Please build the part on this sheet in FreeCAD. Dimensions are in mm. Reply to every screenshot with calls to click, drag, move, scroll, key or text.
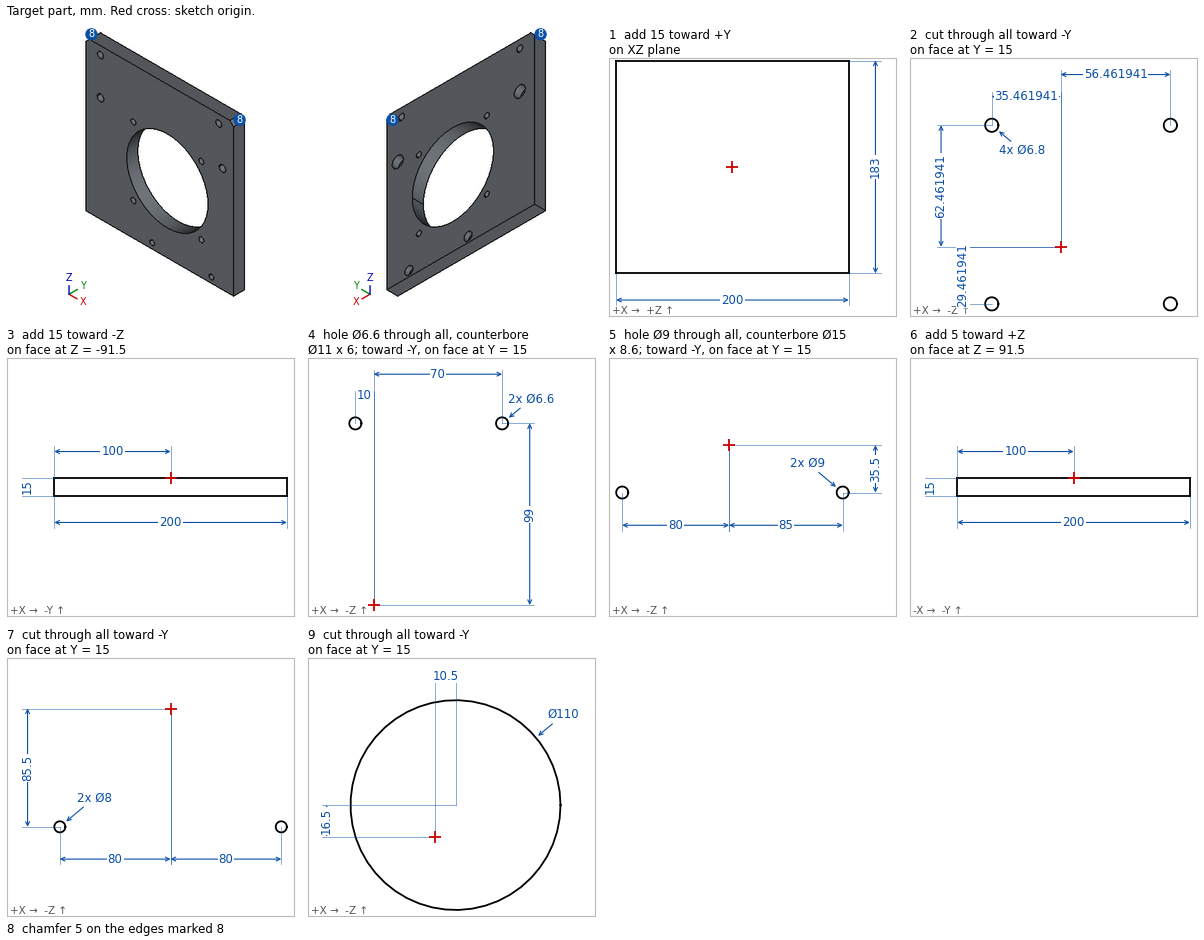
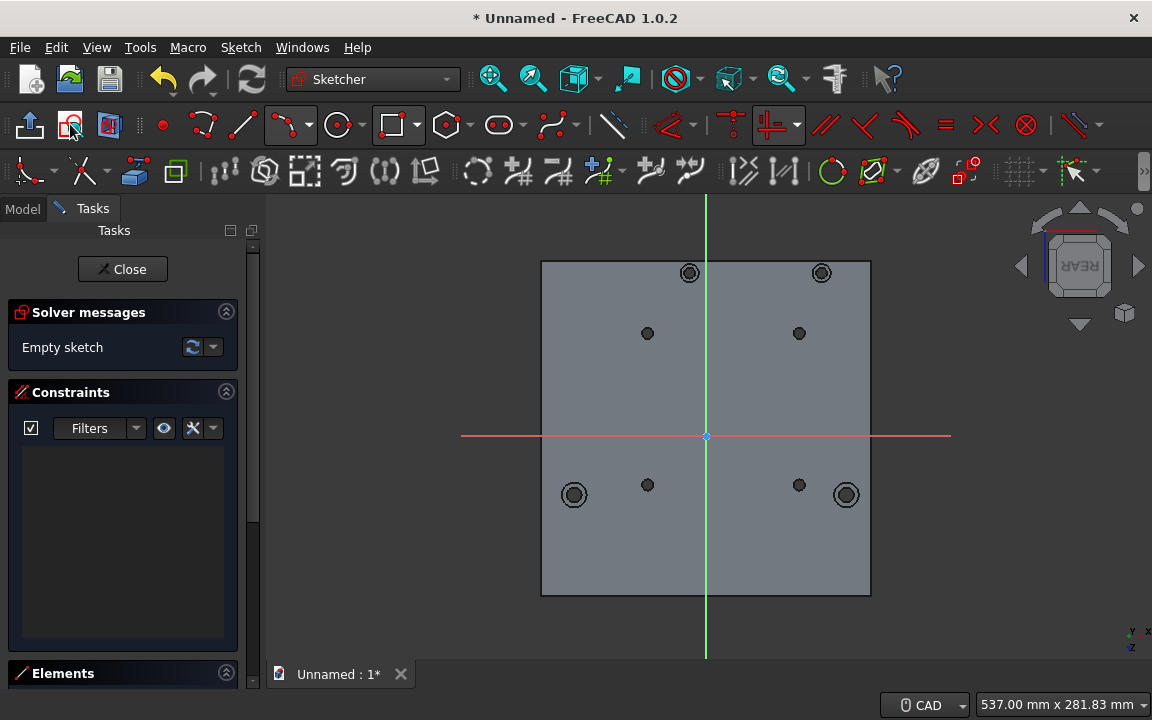
scroll(786, 612, up, 3)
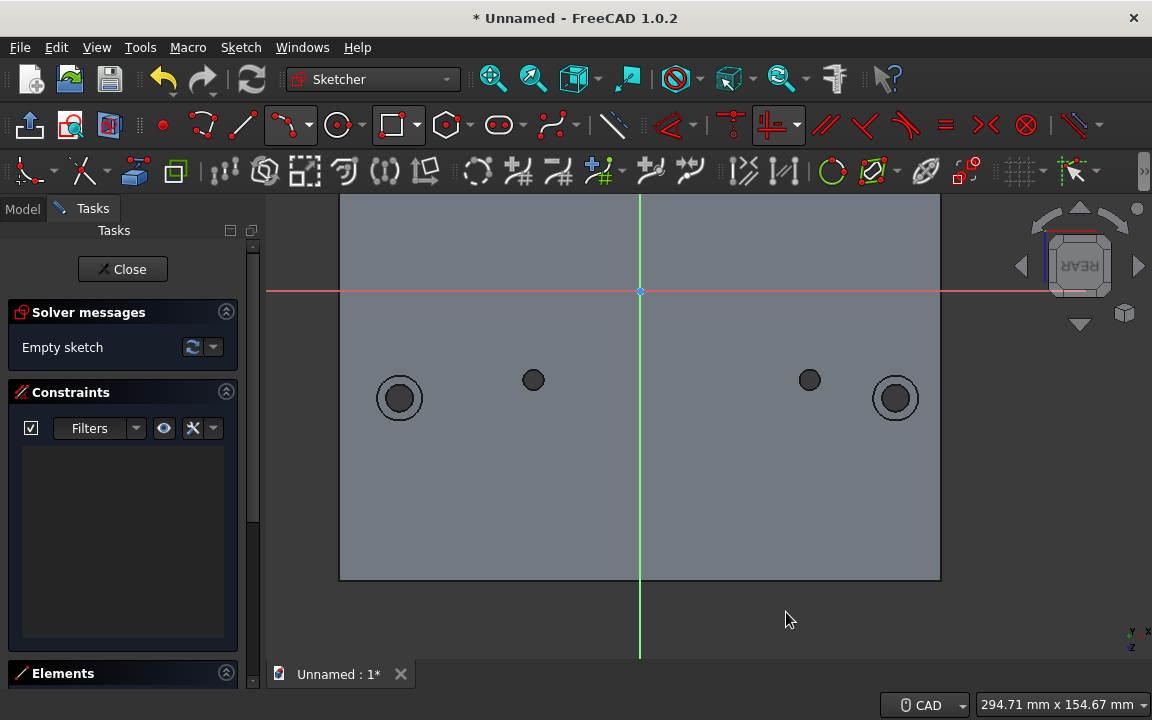
click(338, 126)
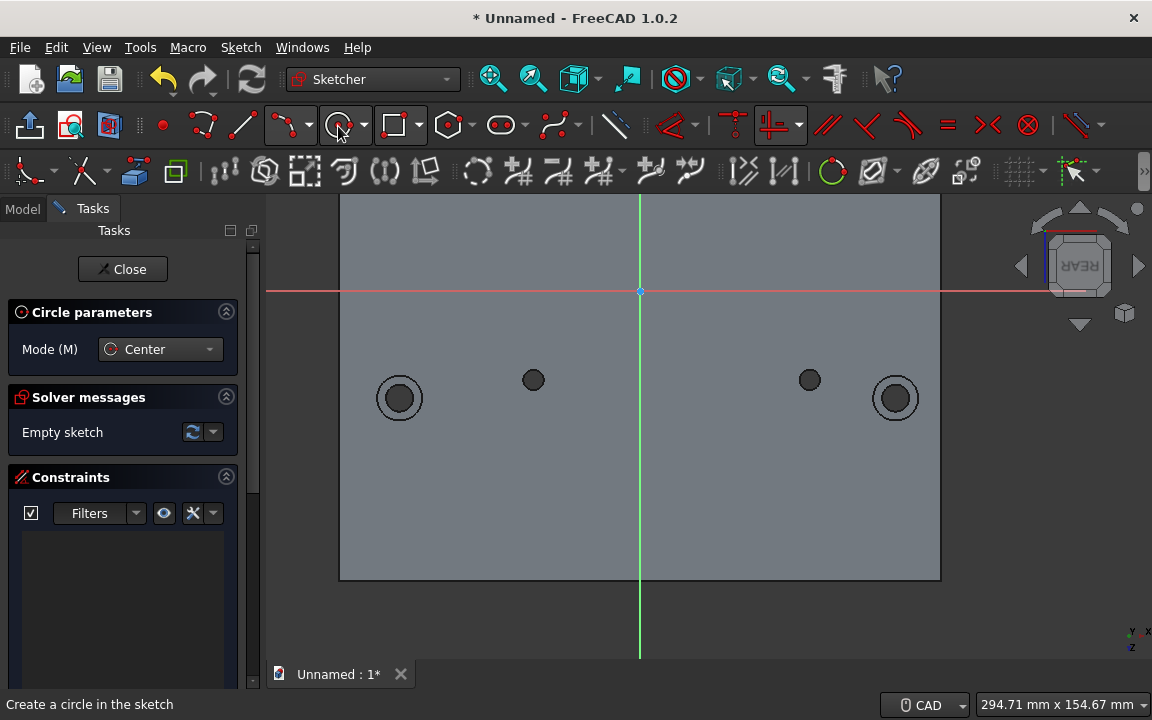
scroll(400, 548, up, 4)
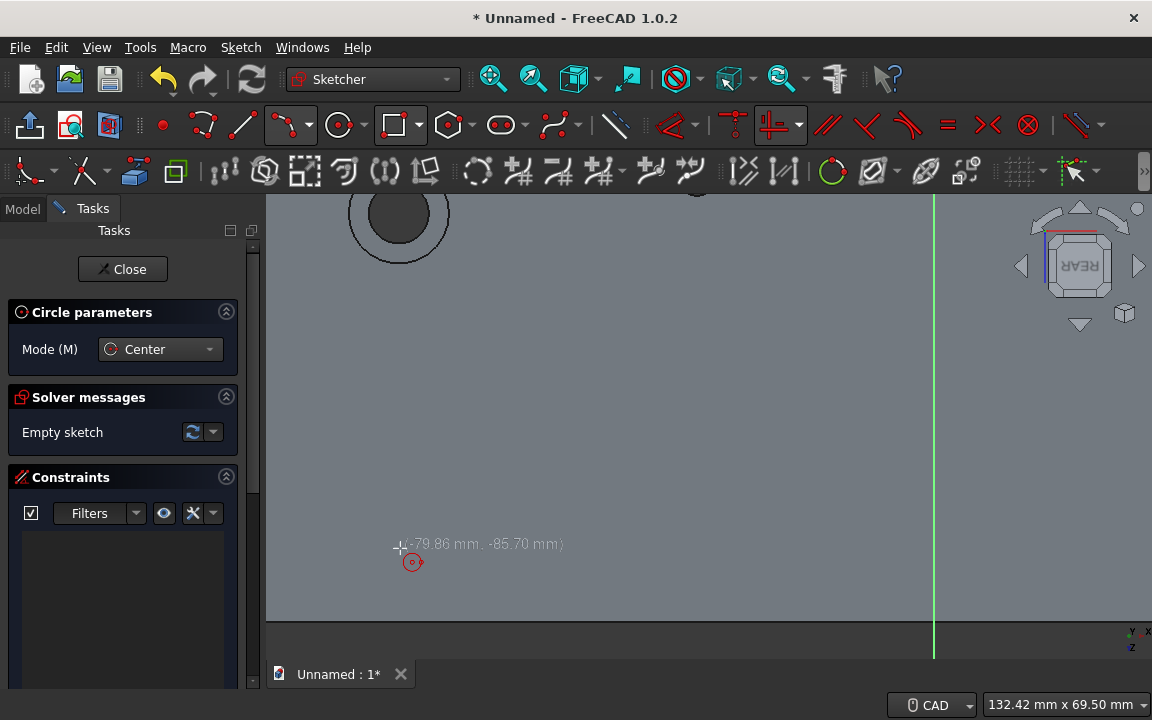
click(399, 548)
click(418, 529)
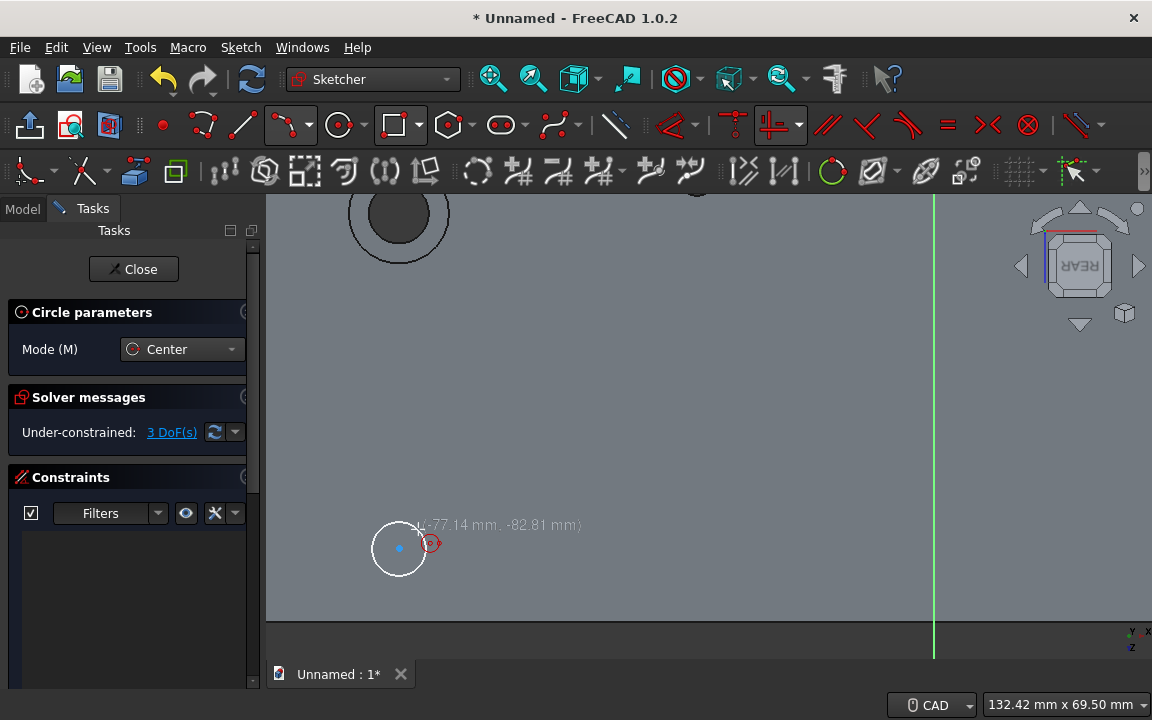
scroll(401, 550, down, 4)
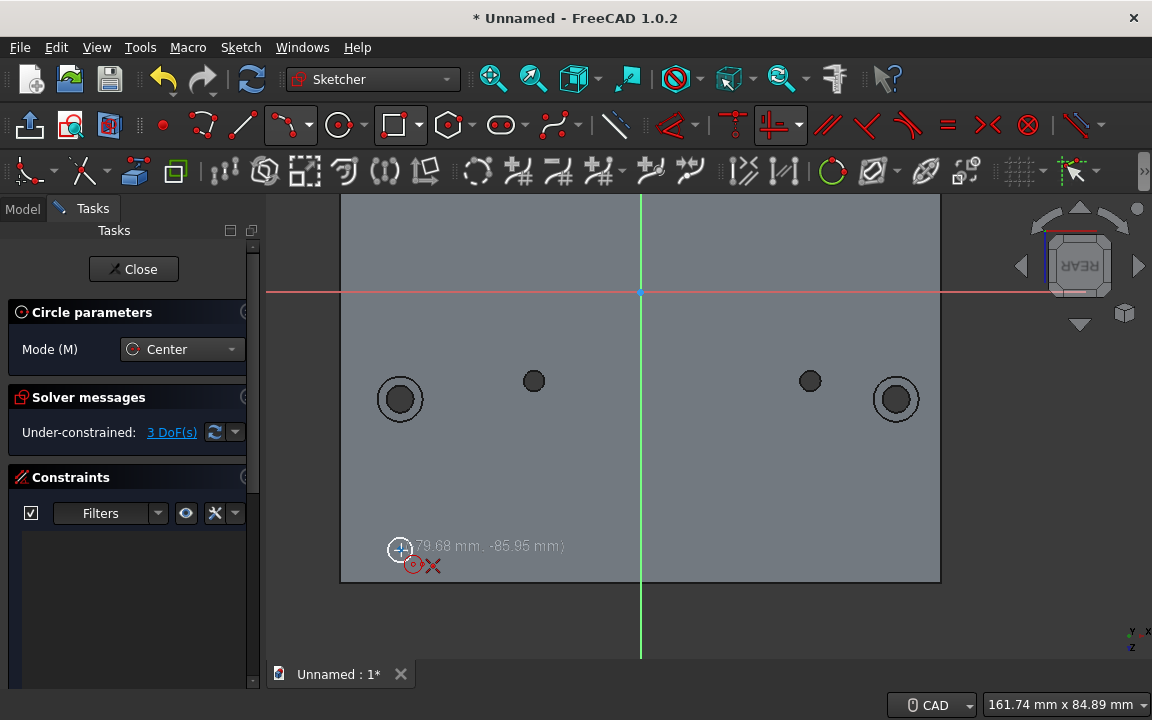
scroll(881, 550, up, 4)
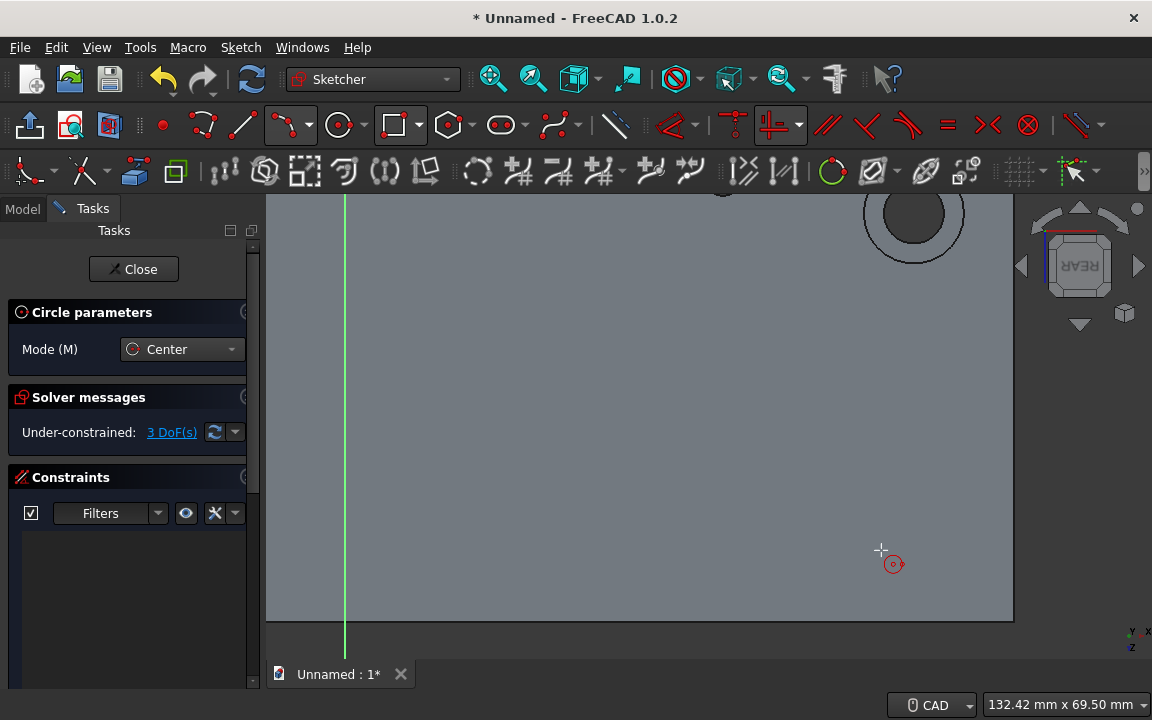
click(880, 548)
click(899, 529)
key(Escape)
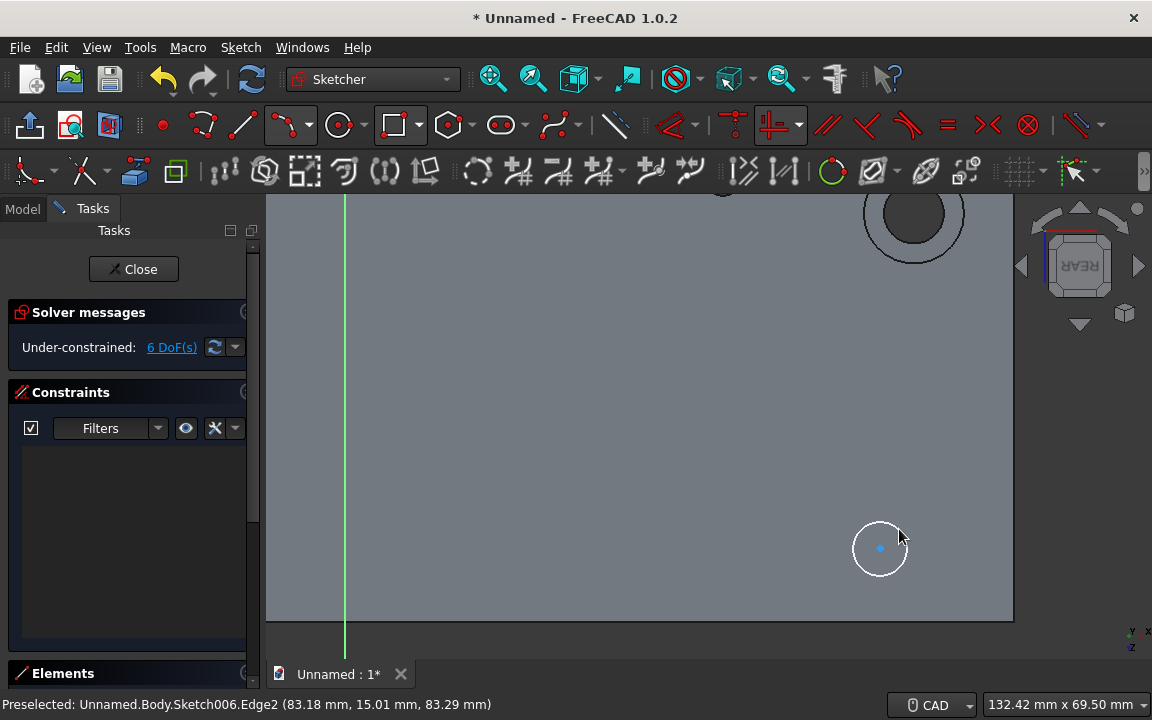
scroll(881, 550, down, 4)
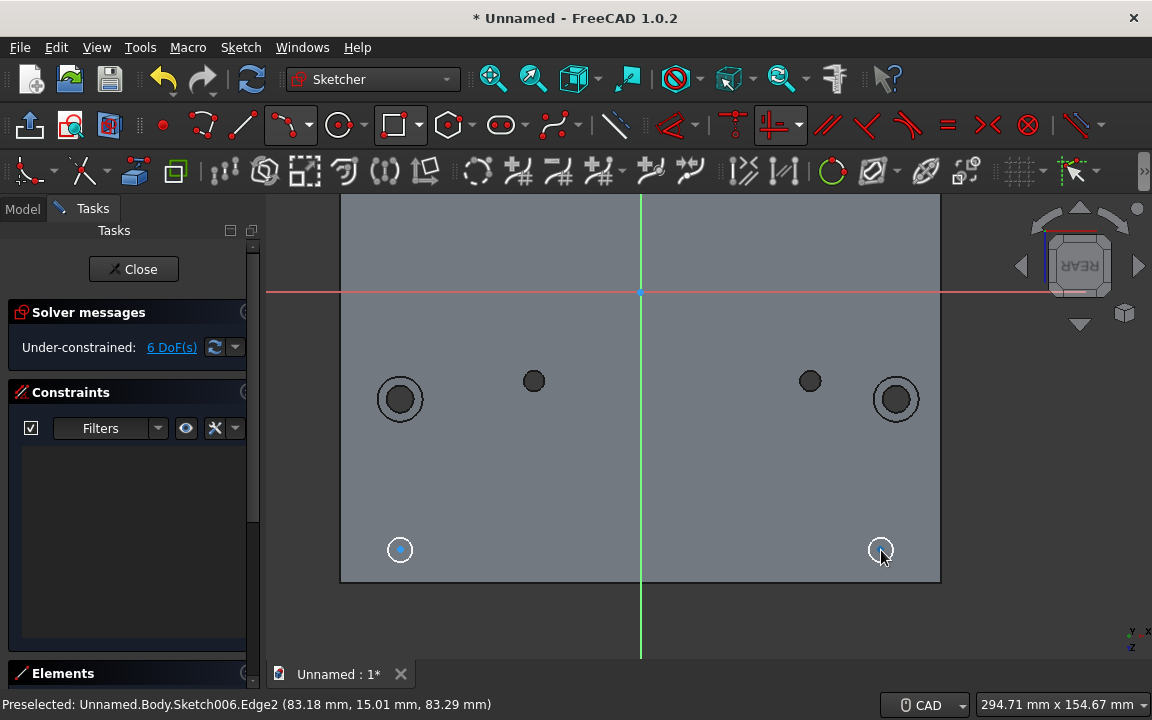
click(409, 541)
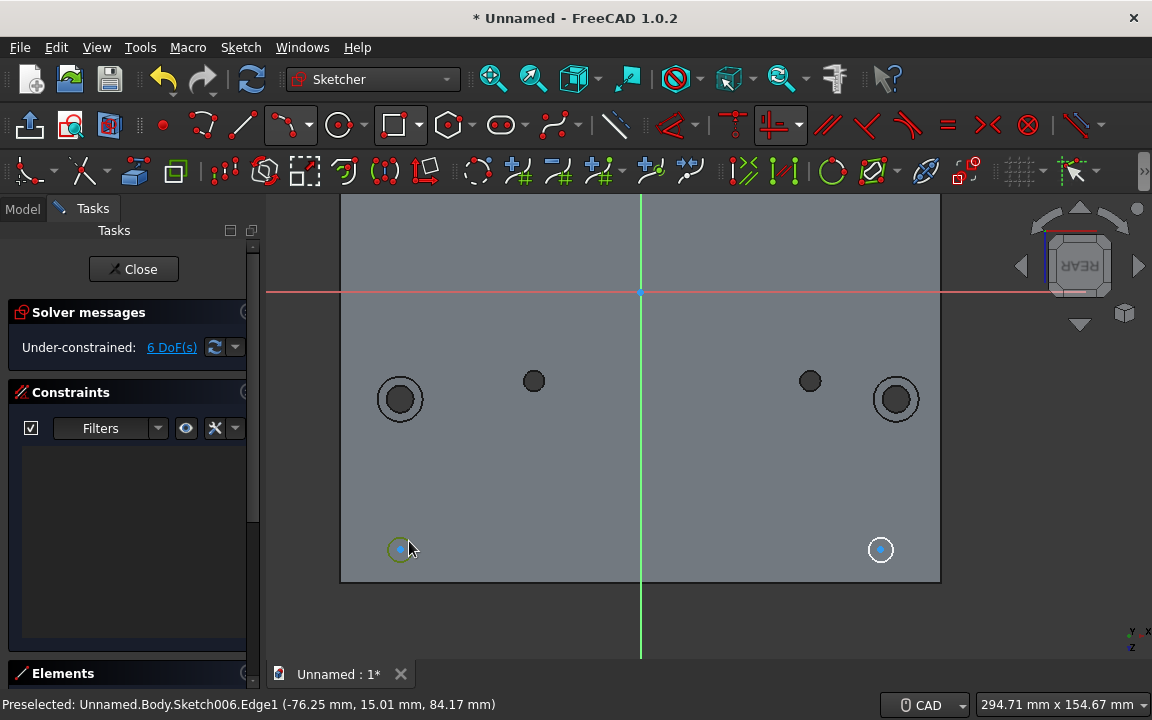
click(889, 541)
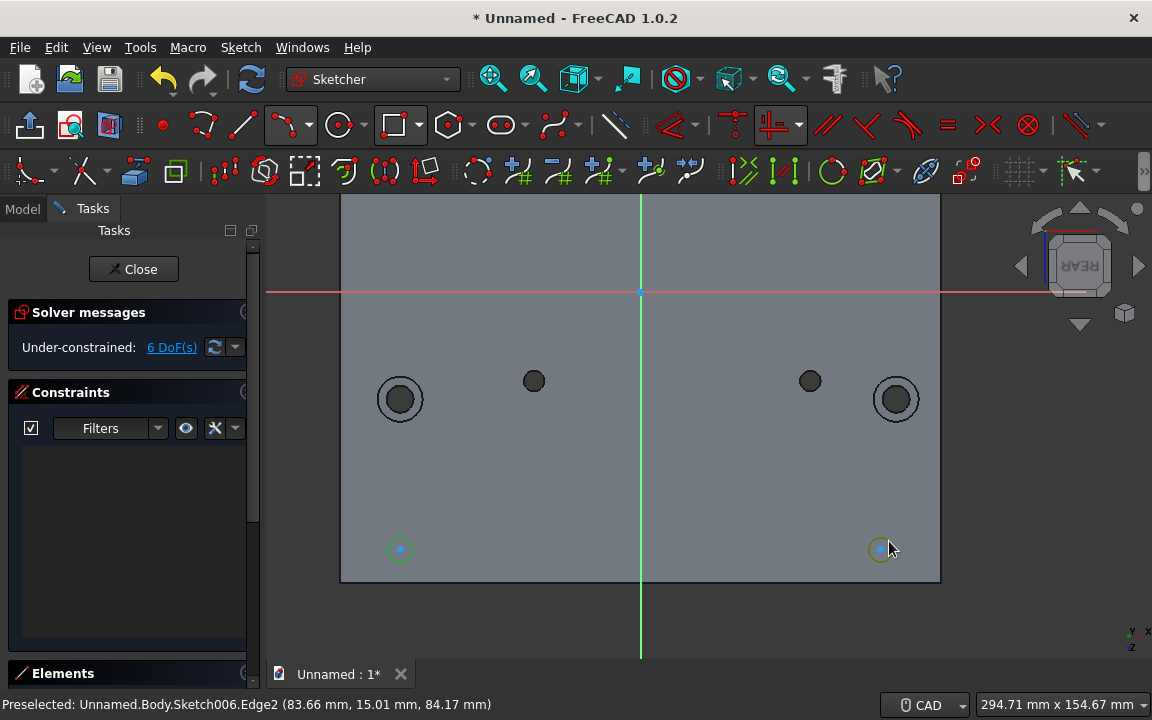
click(948, 126)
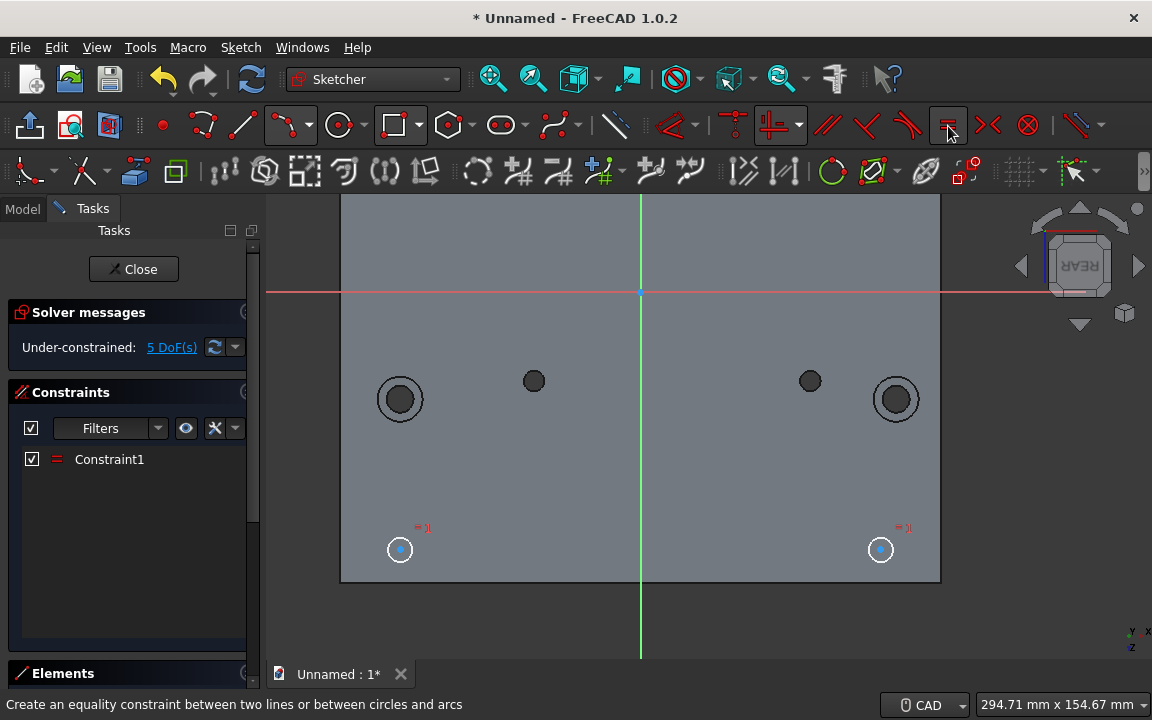
click(400, 550)